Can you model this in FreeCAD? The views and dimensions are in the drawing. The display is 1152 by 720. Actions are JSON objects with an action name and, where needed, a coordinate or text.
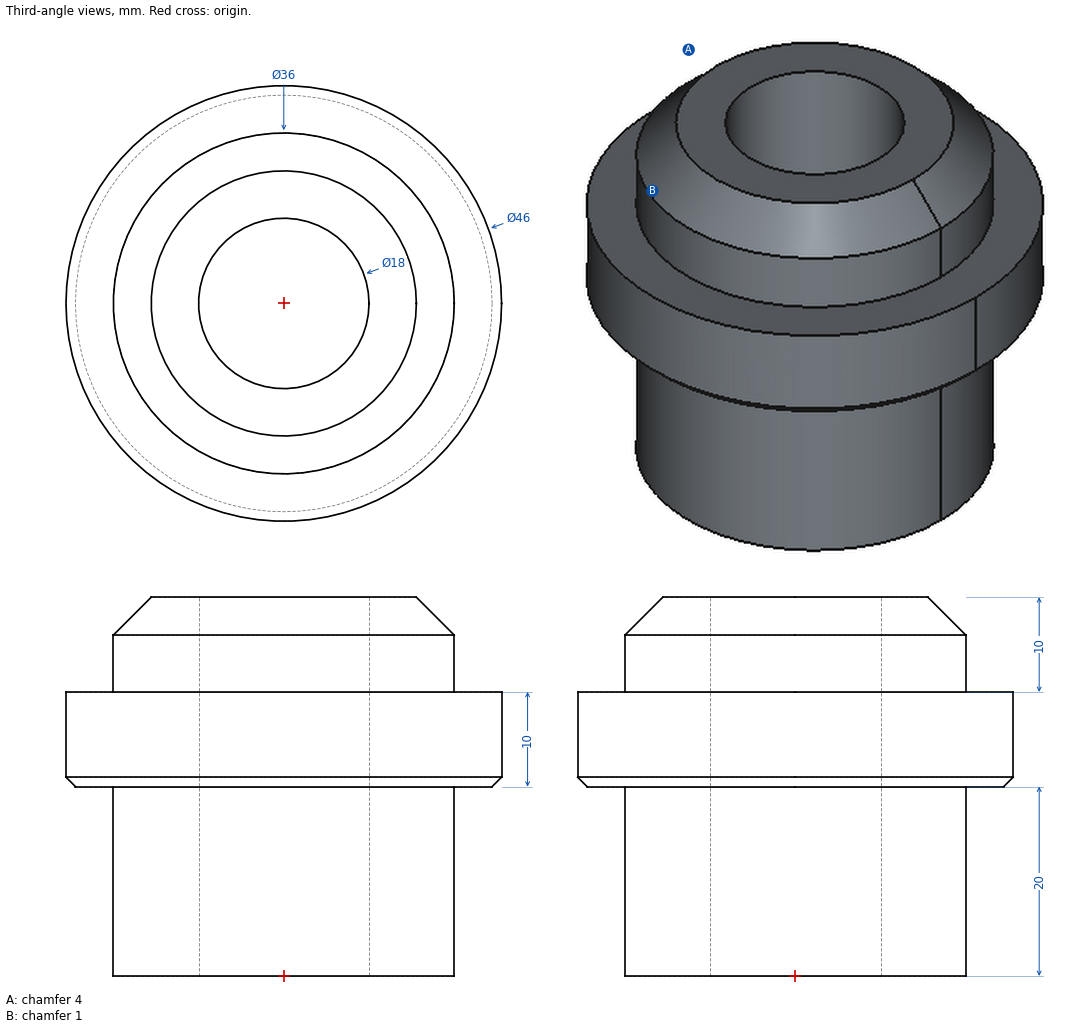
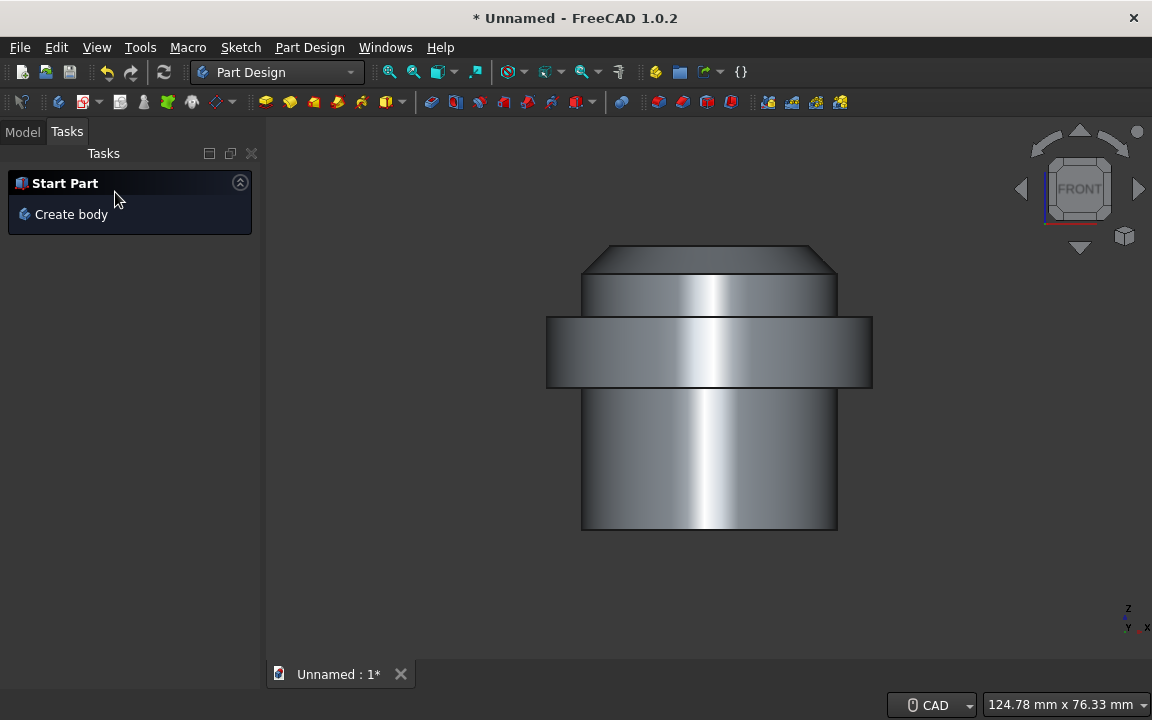
{"action": "left_click", "coordinate": [577, 387]}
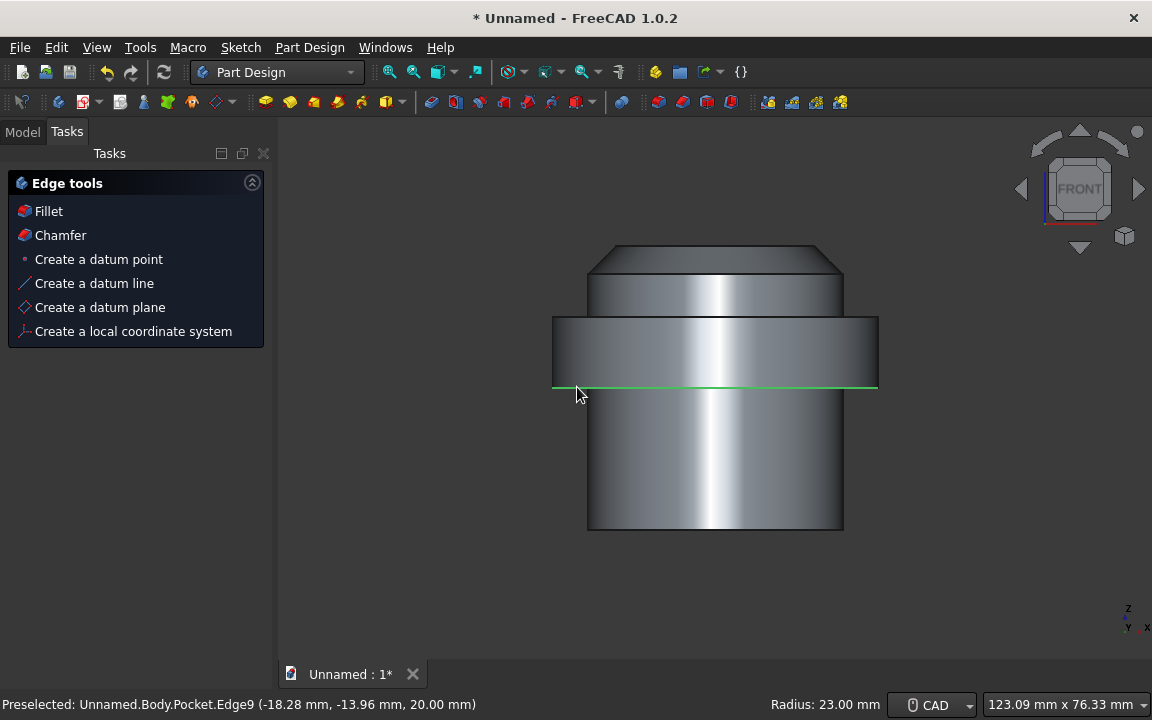
{"action": "left_click", "coordinate": [684, 102]}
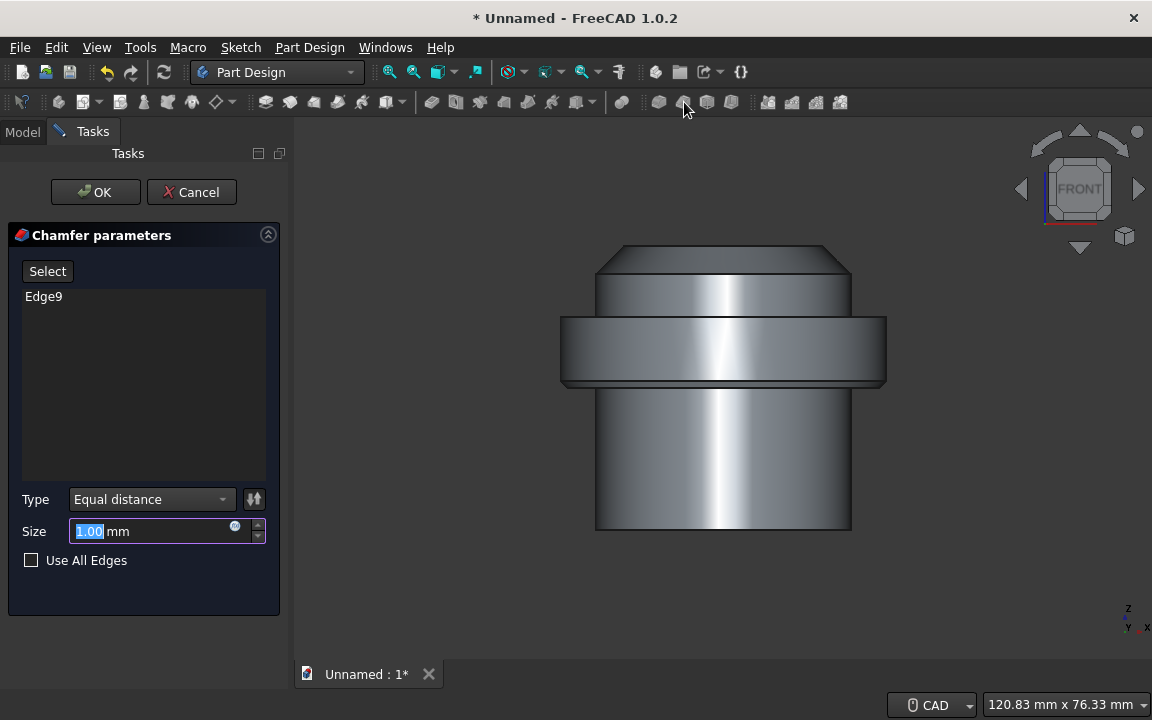
{"action": "type", "text": "1"}
{"action": "key", "text": "Tab"}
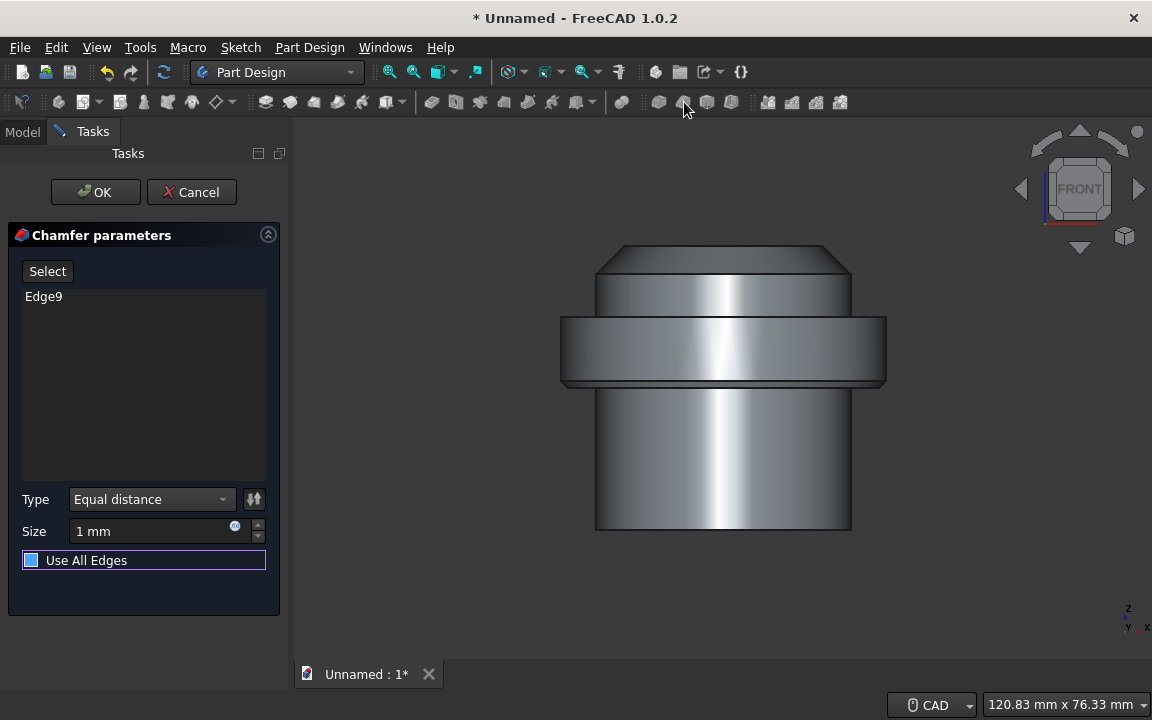
{"action": "left_click", "coordinate": [96, 192]}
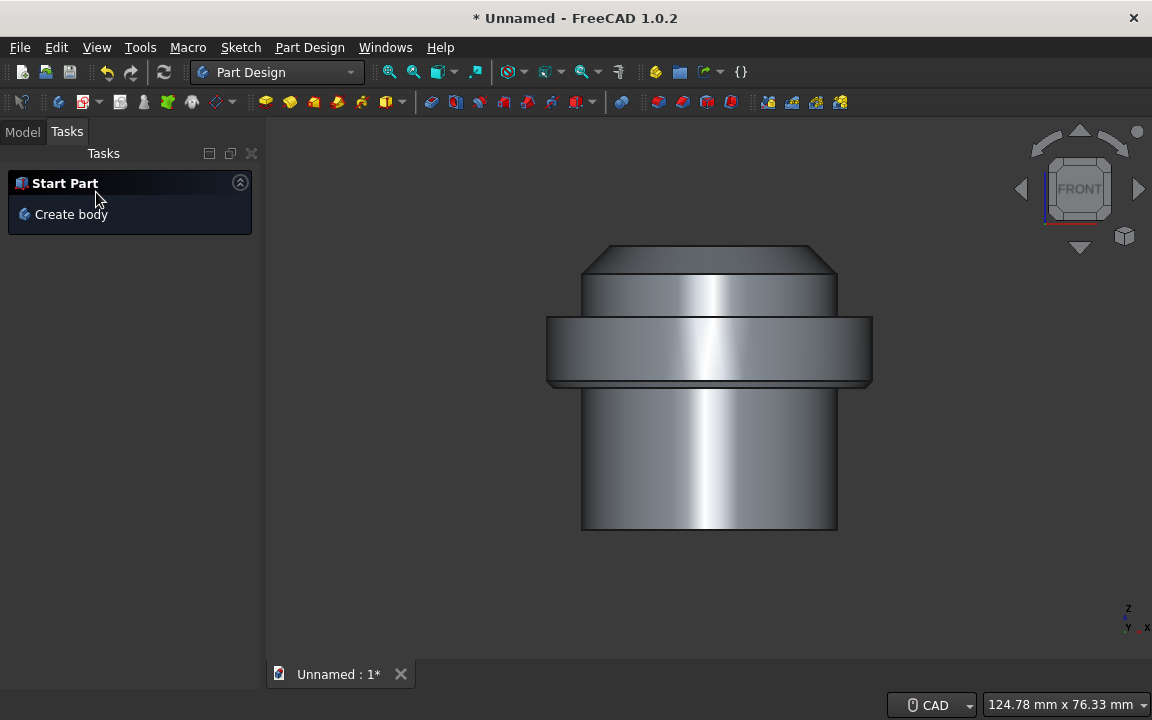
{"action": "key", "text": "0"}